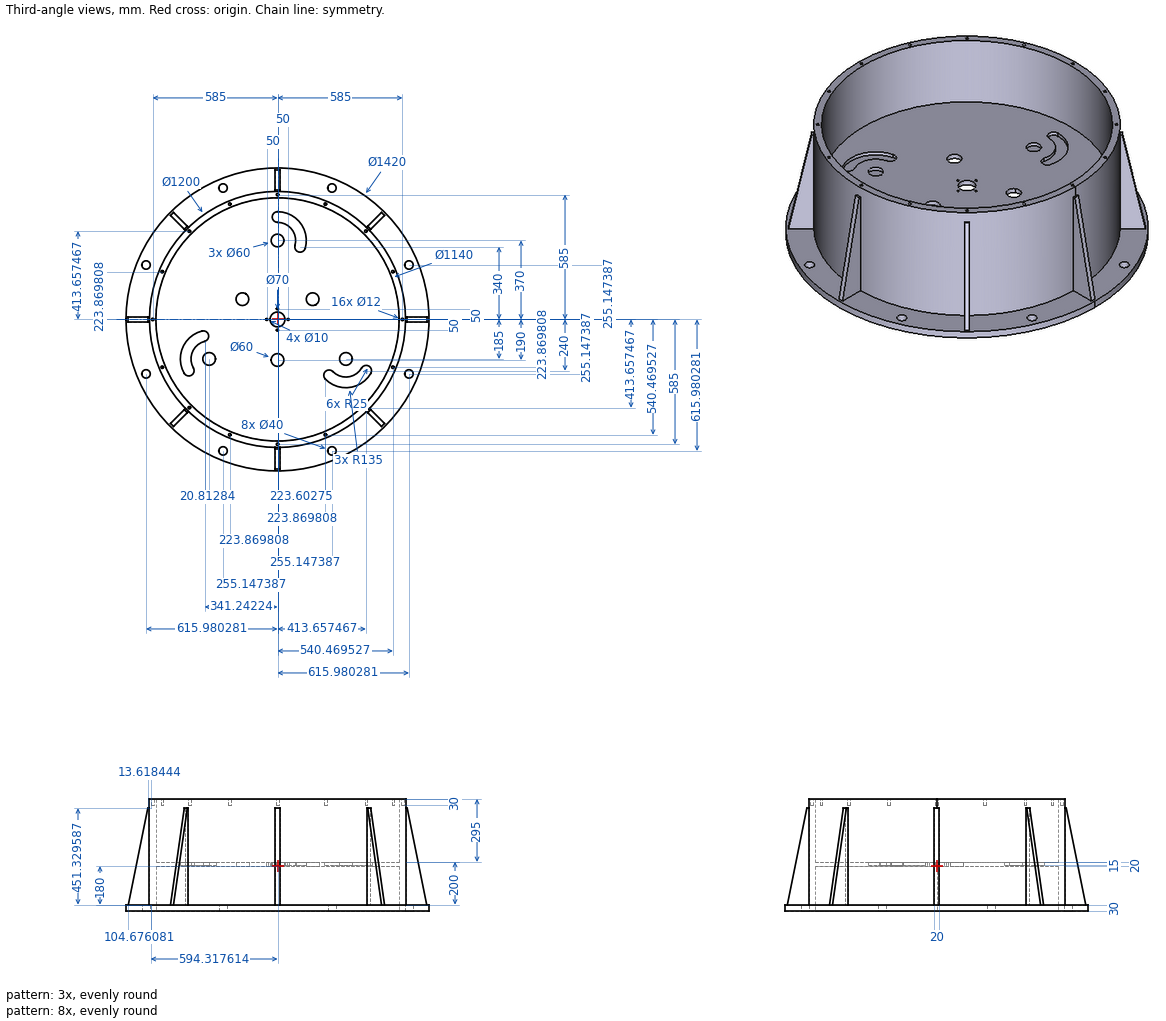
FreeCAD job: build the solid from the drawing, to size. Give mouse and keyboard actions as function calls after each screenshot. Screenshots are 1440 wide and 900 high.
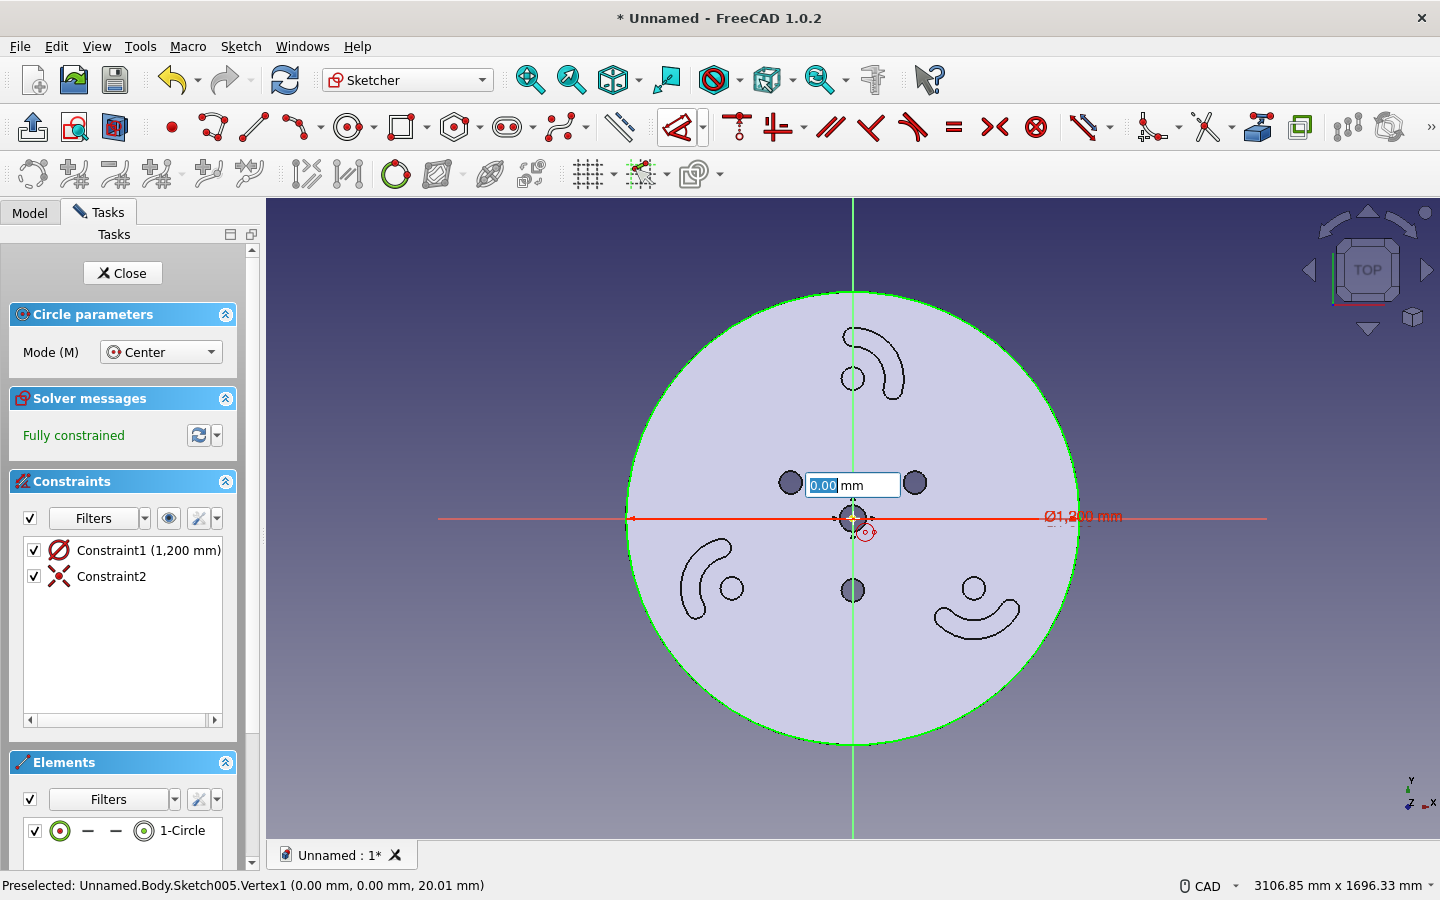
scroll(1005, 366, up, 2)
move(1005, 366)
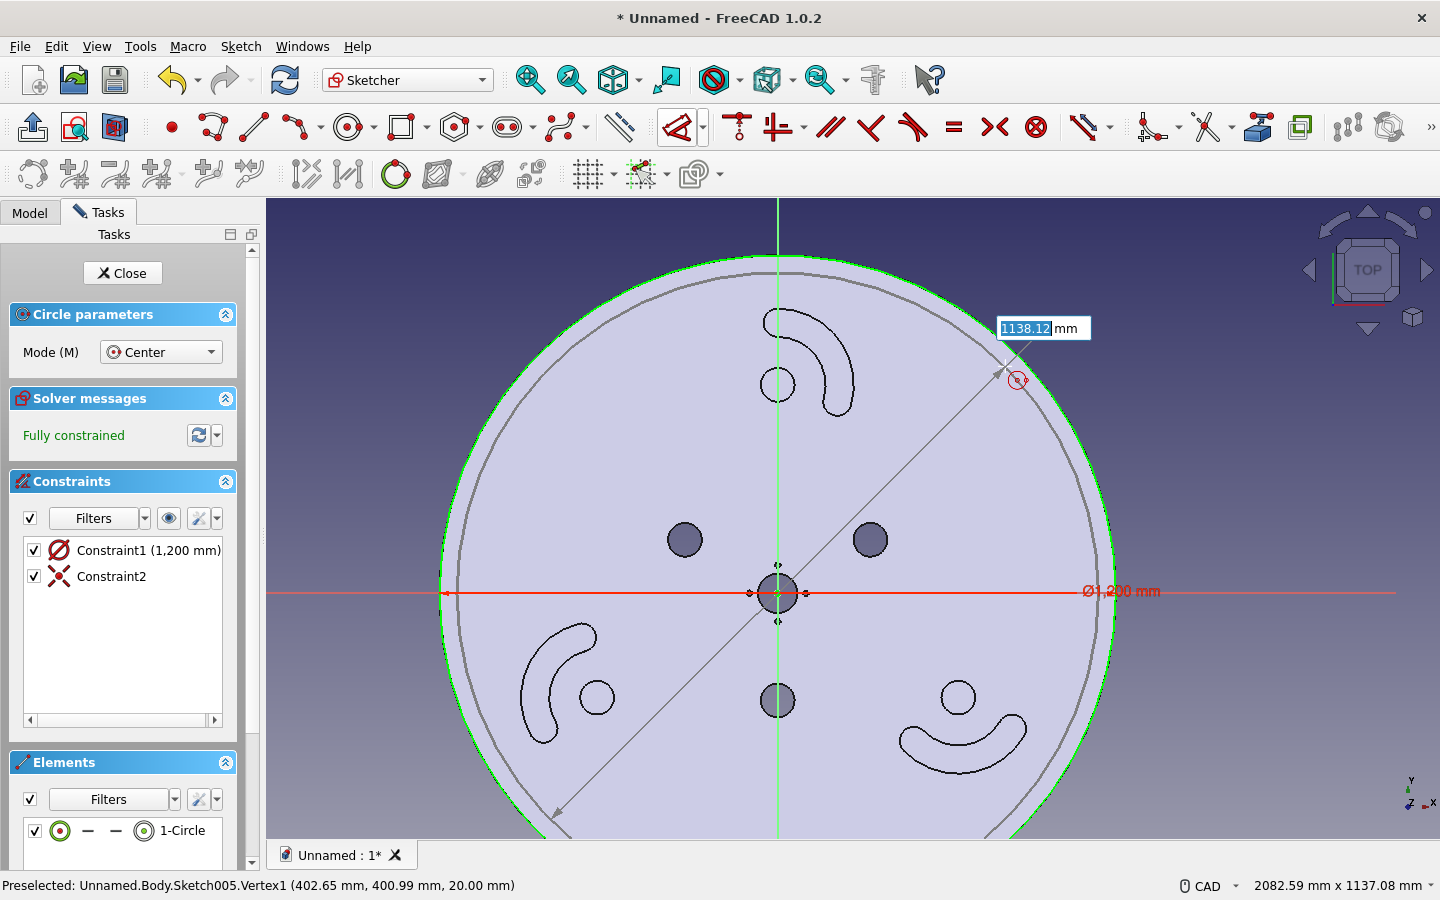
text(1140)
key(Return)
key(Escape)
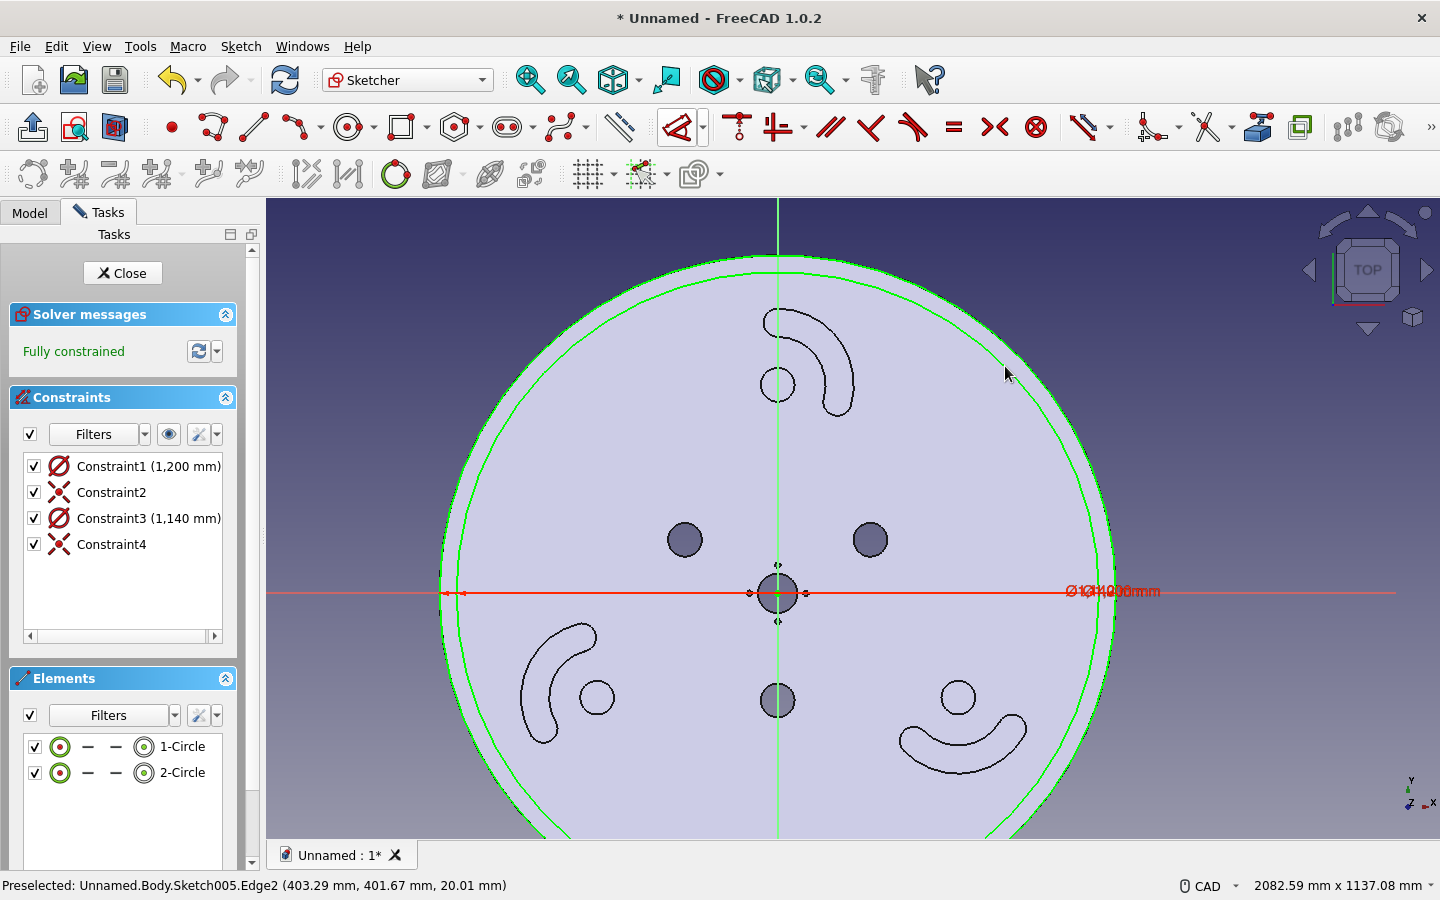
click(123, 273)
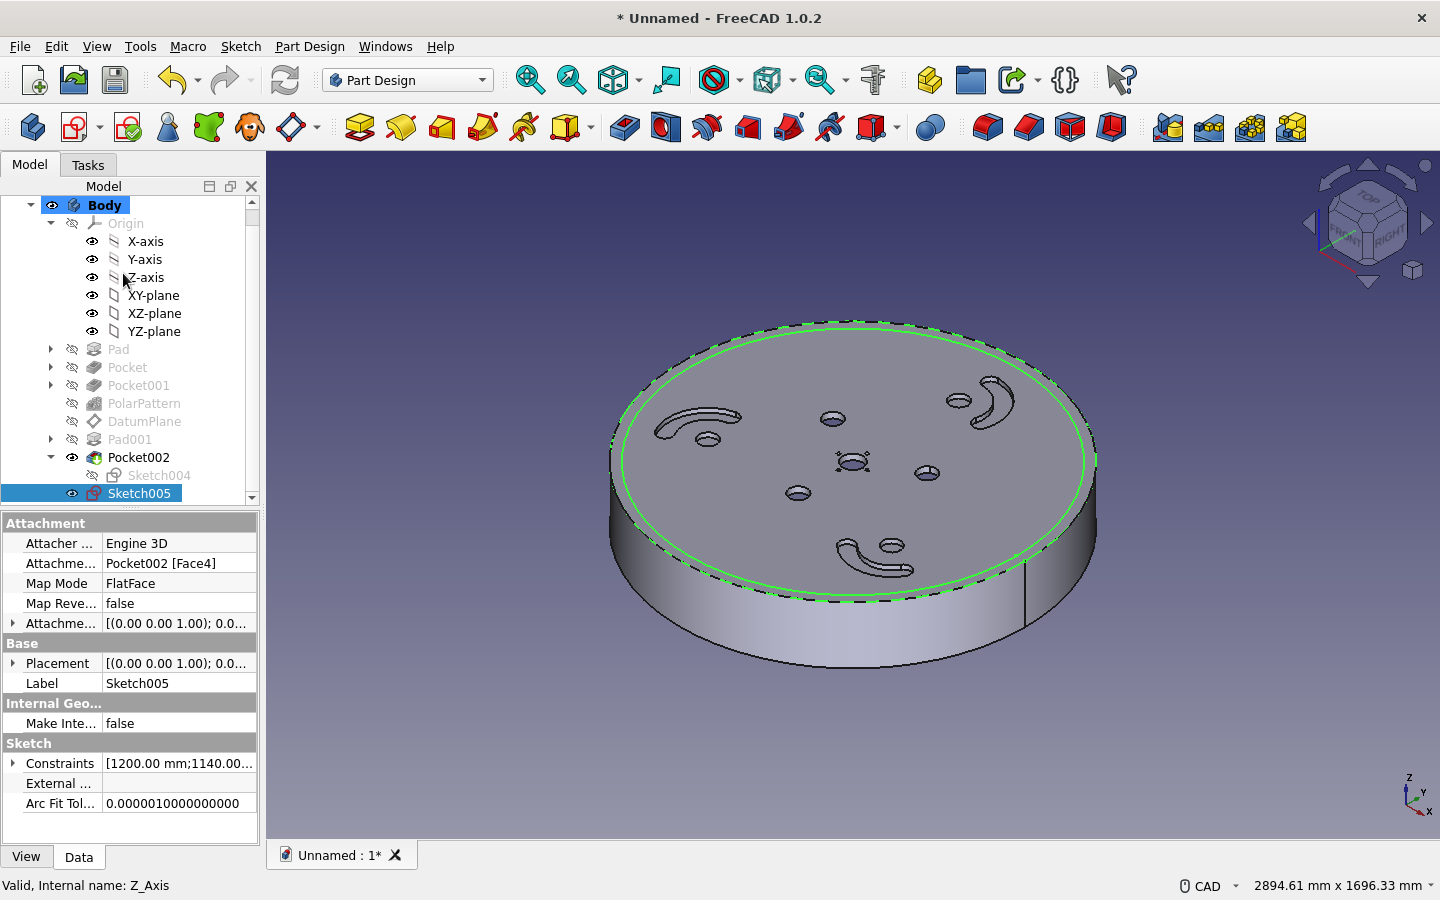
click(360, 128)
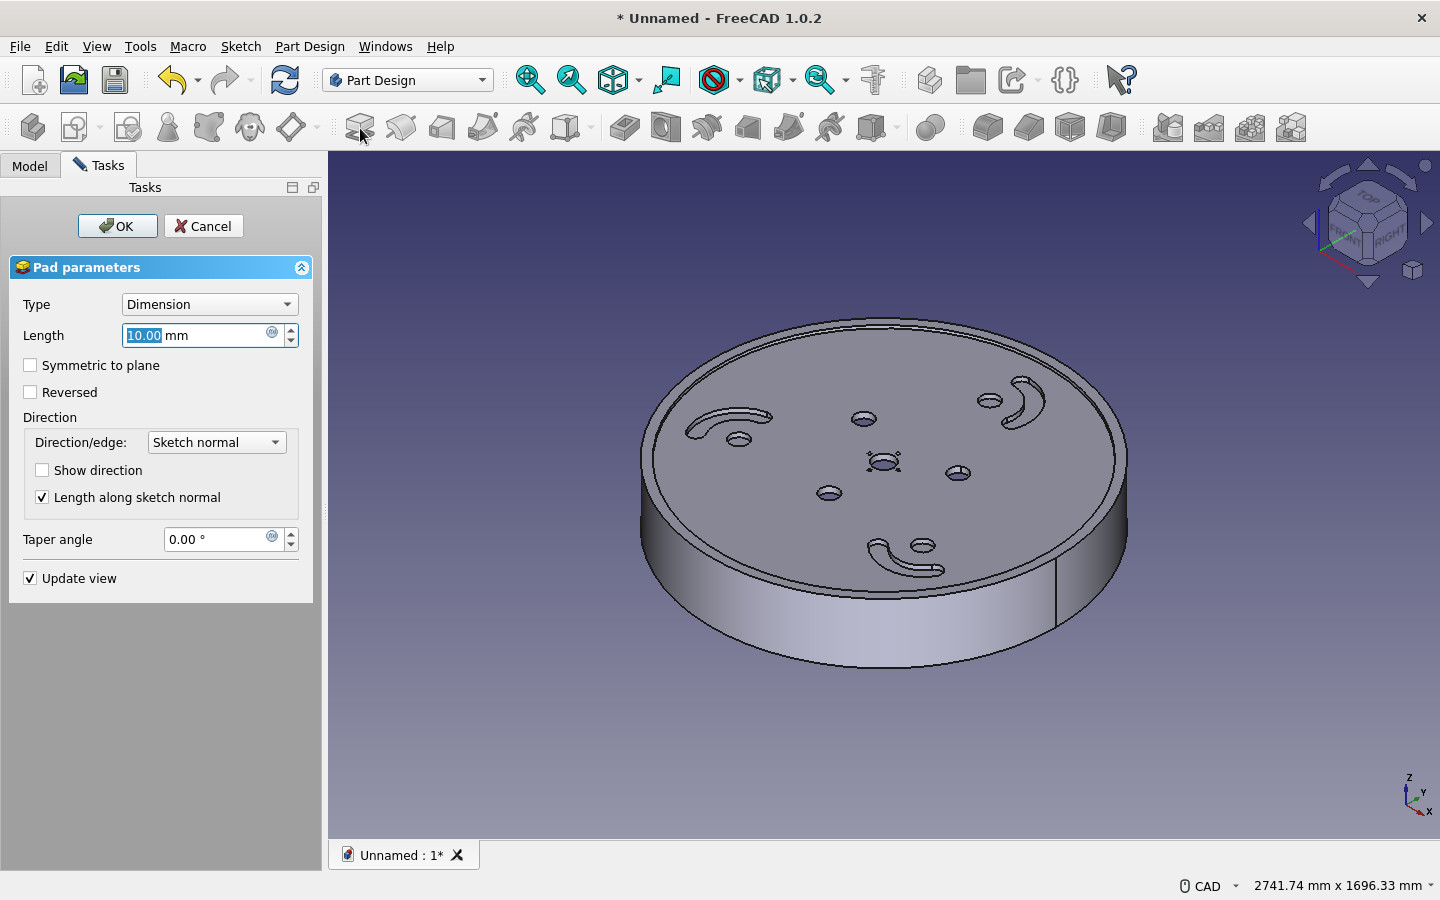
text(295)
key(Tab)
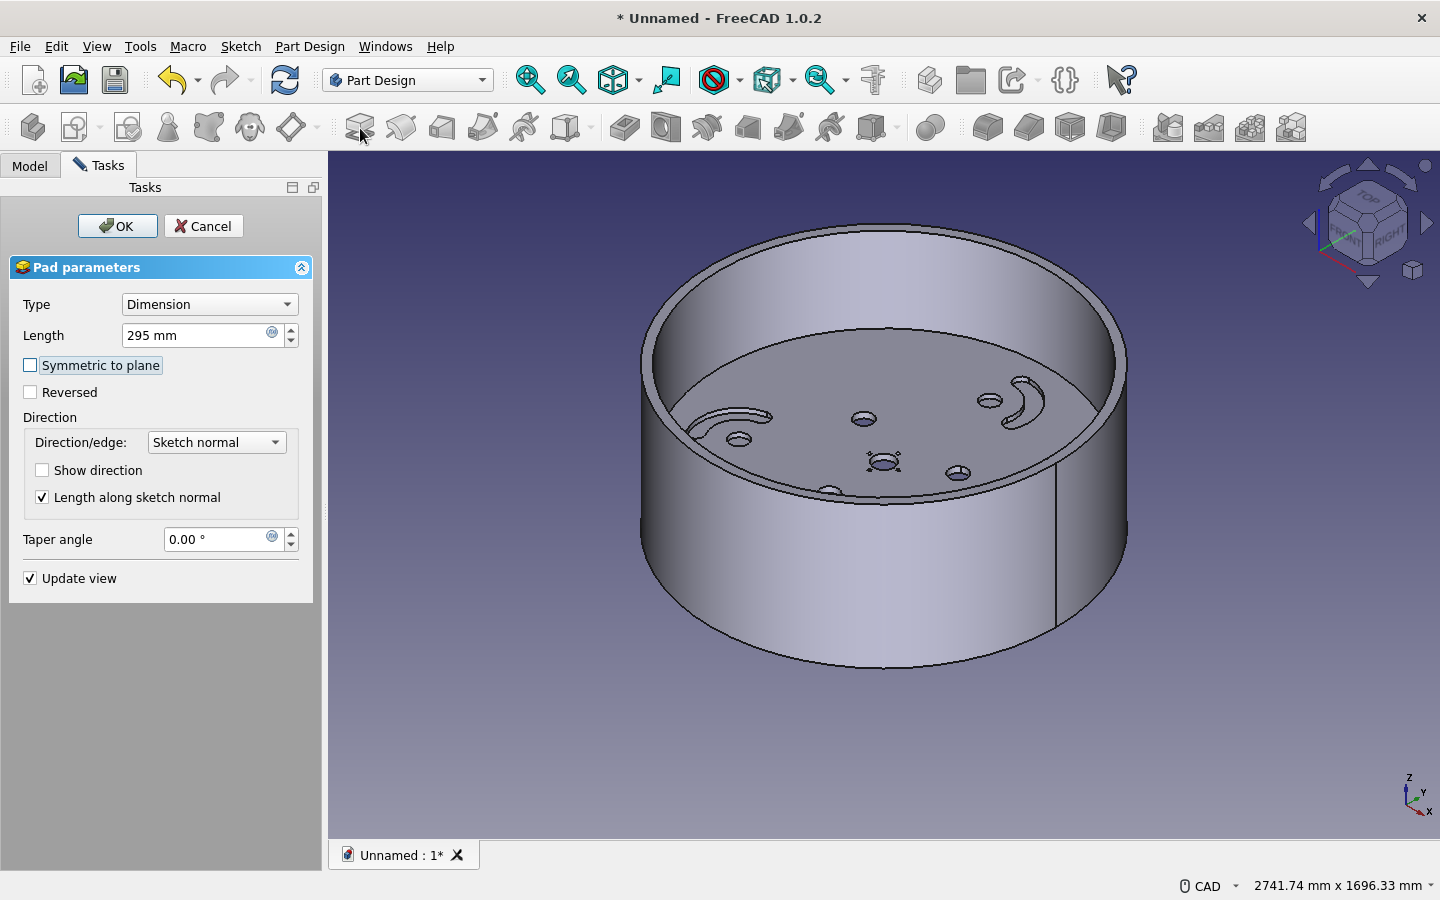
click(118, 226)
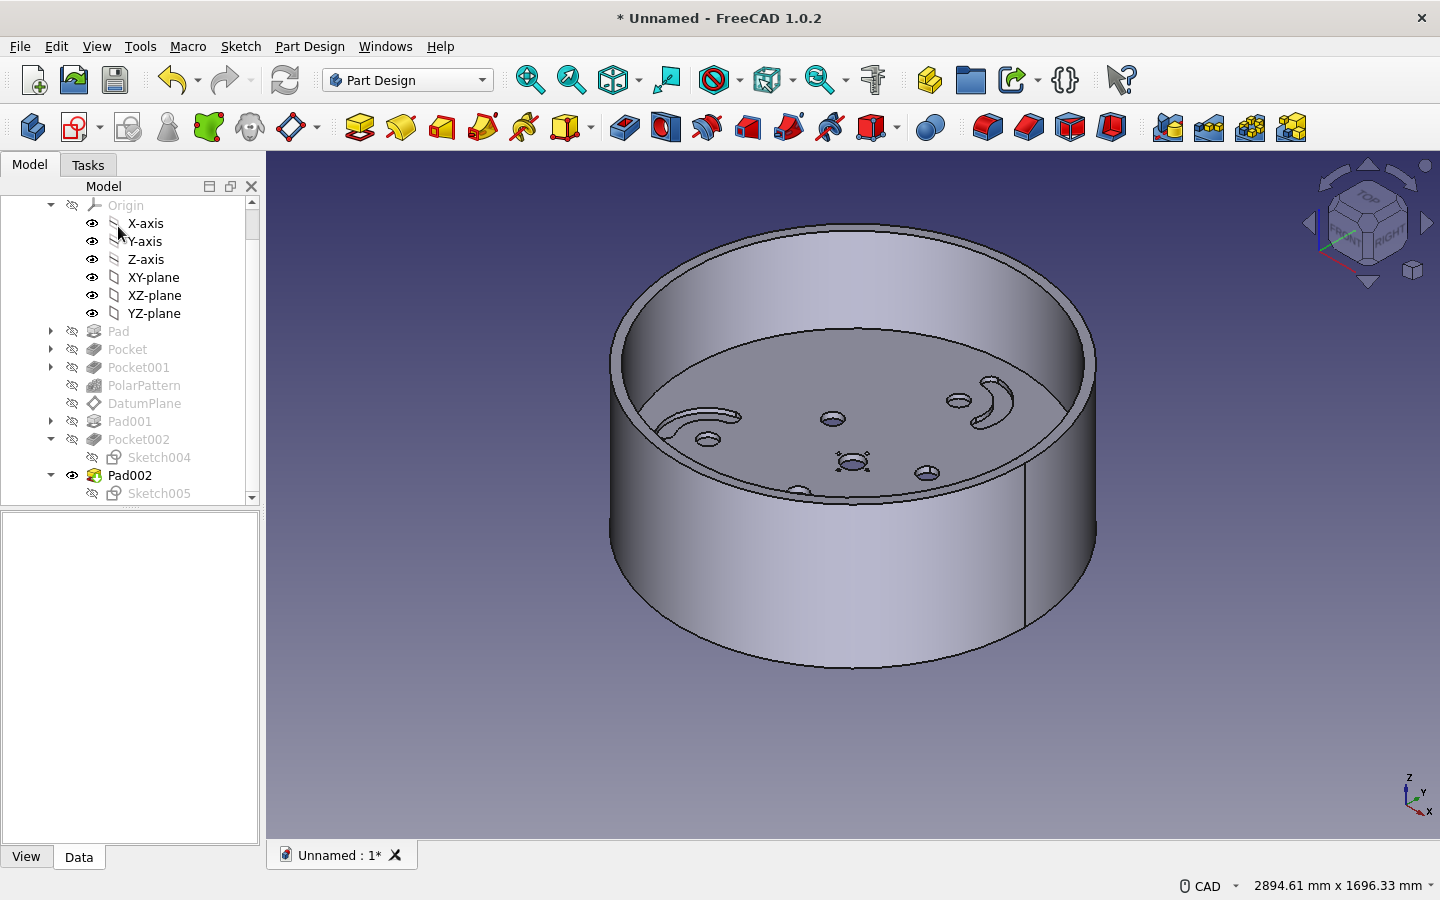
click(137, 277)